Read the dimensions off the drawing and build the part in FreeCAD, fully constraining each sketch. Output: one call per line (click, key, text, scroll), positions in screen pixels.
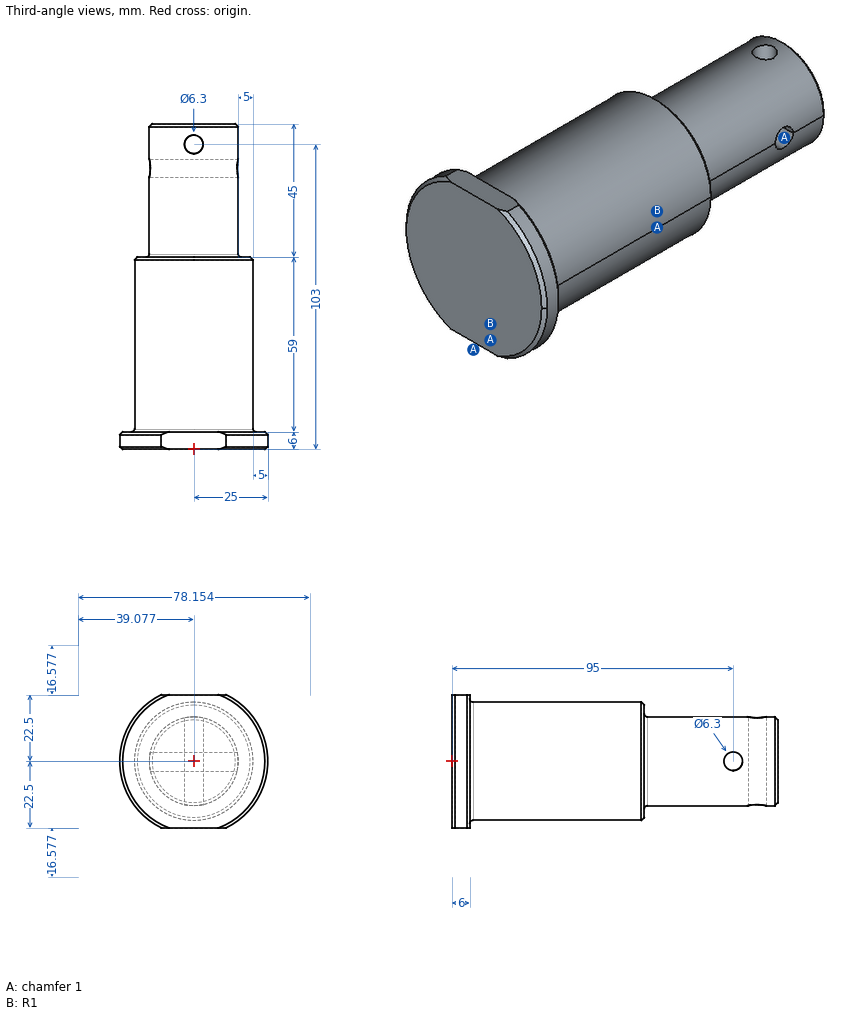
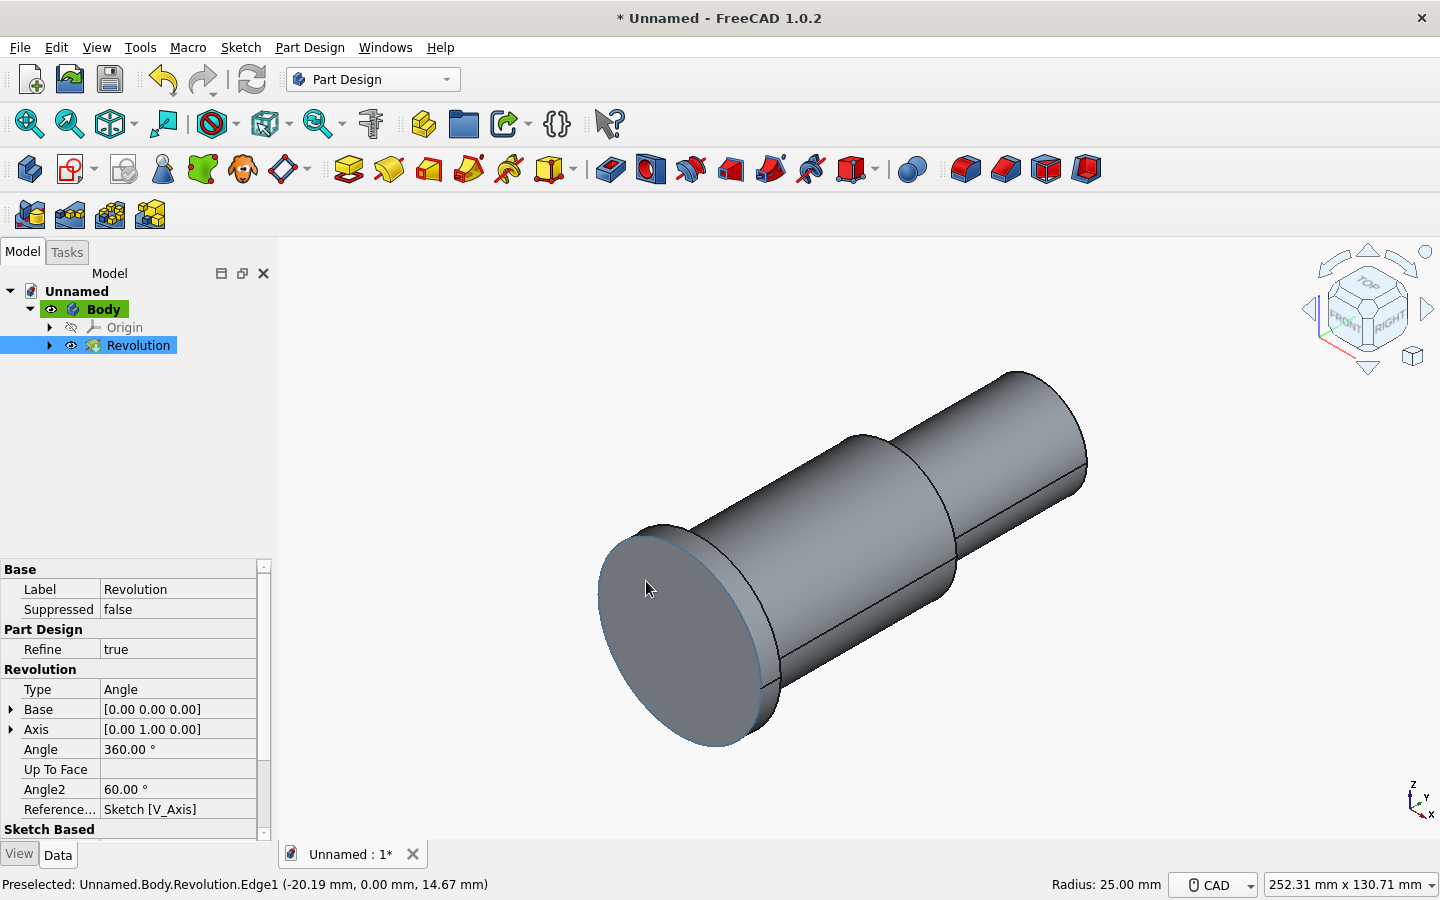
key(2)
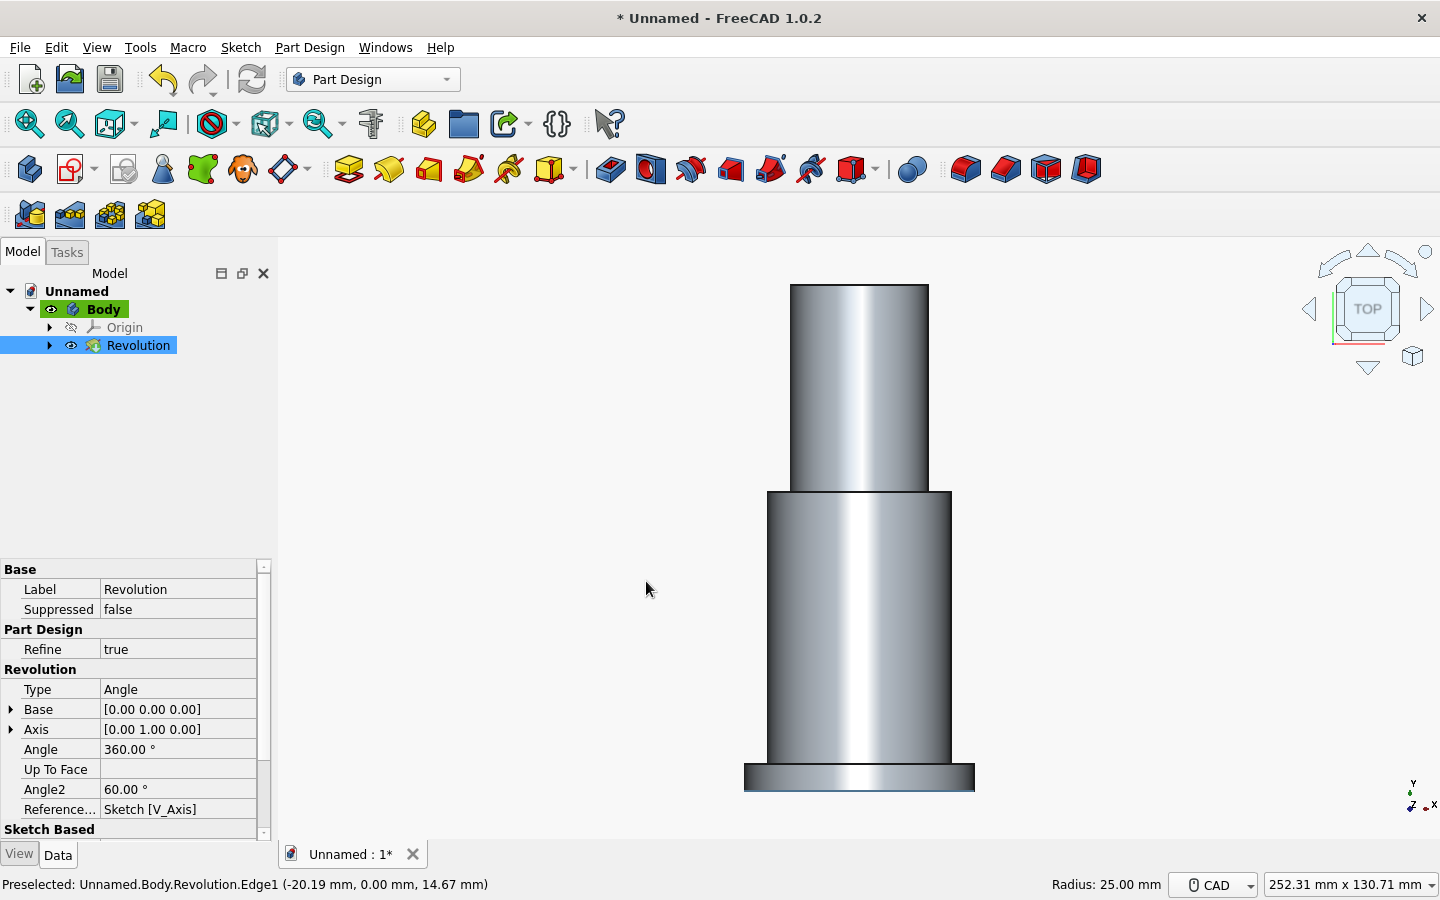
click(803, 284, ctrl)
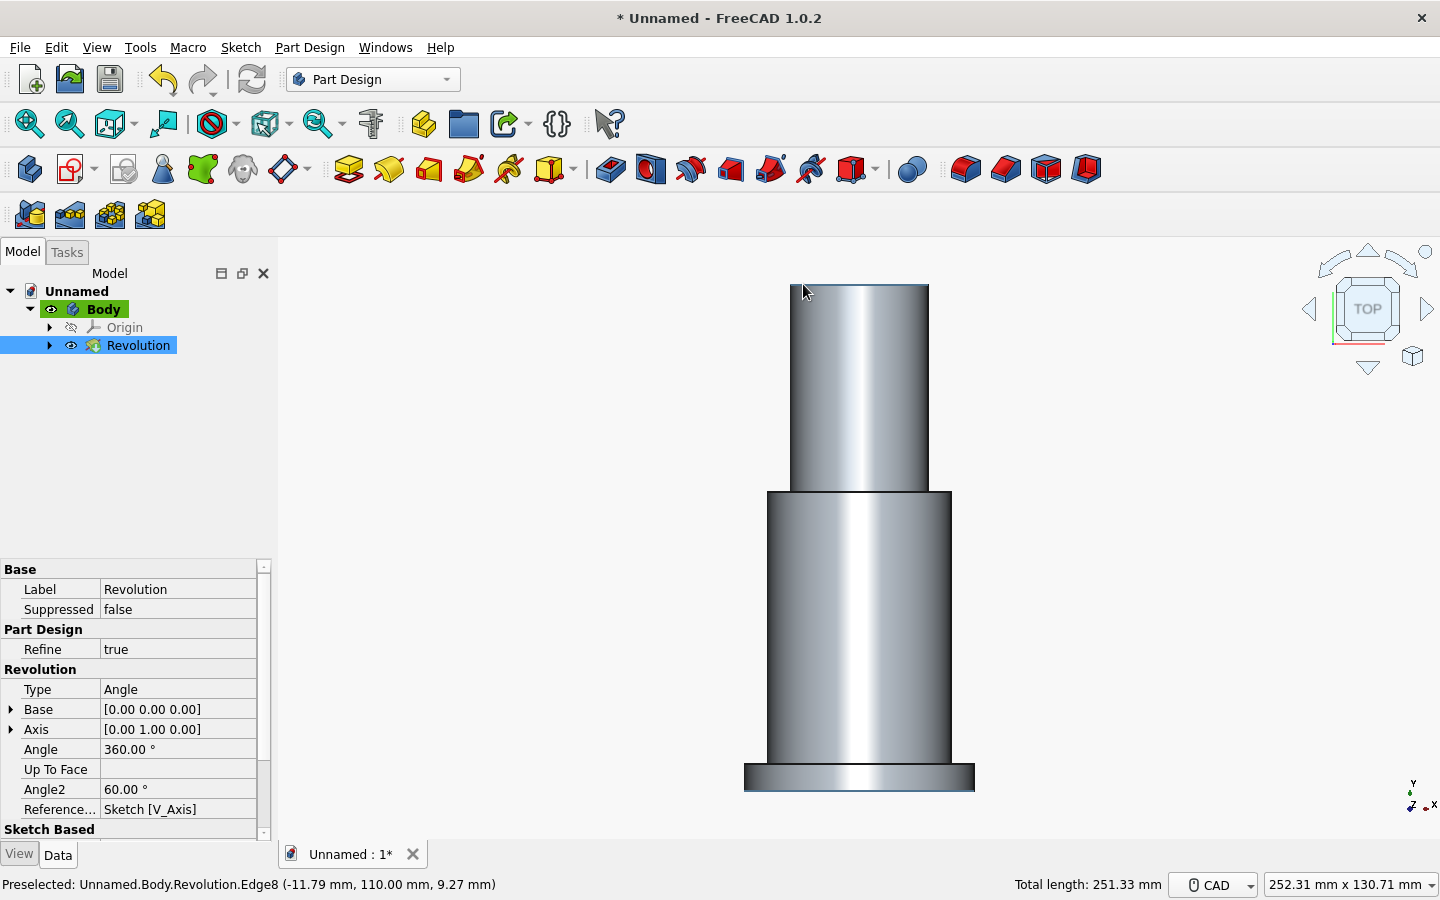
click(784, 491, ctrl)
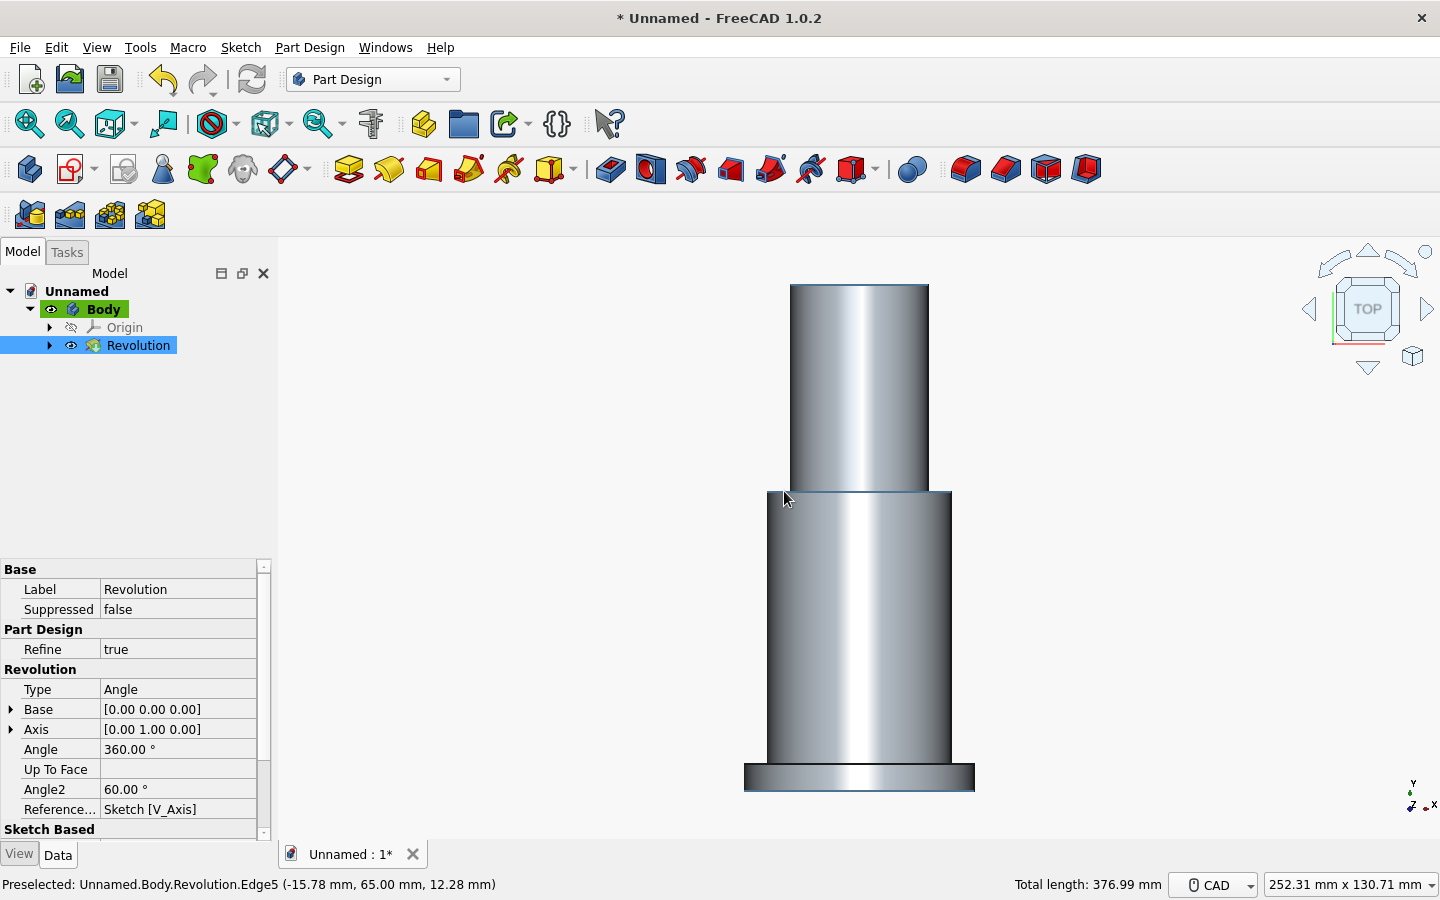
click(766, 763, ctrl)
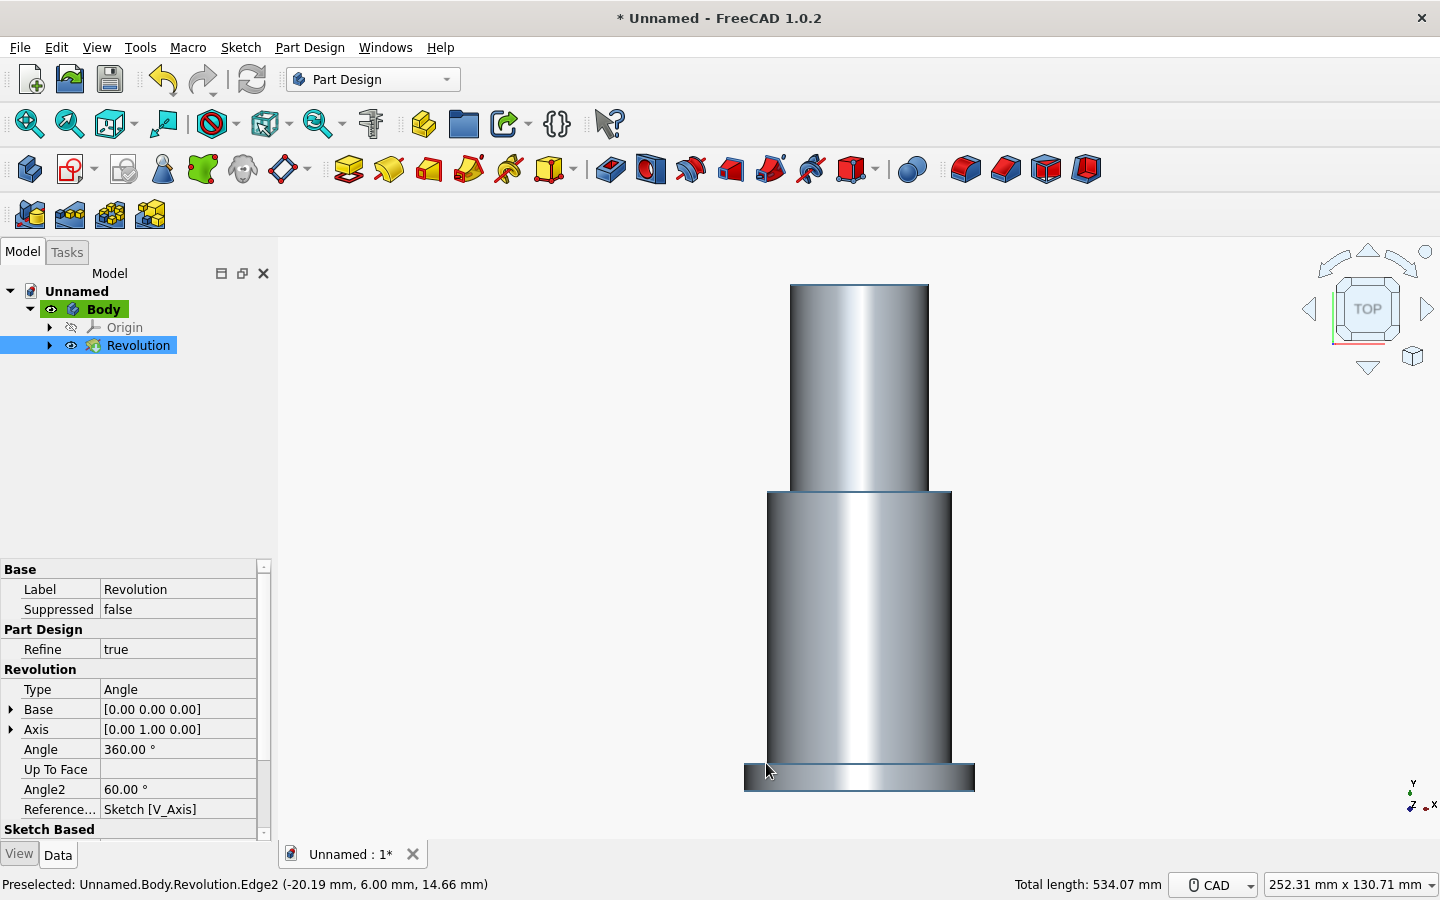
click(1006, 170)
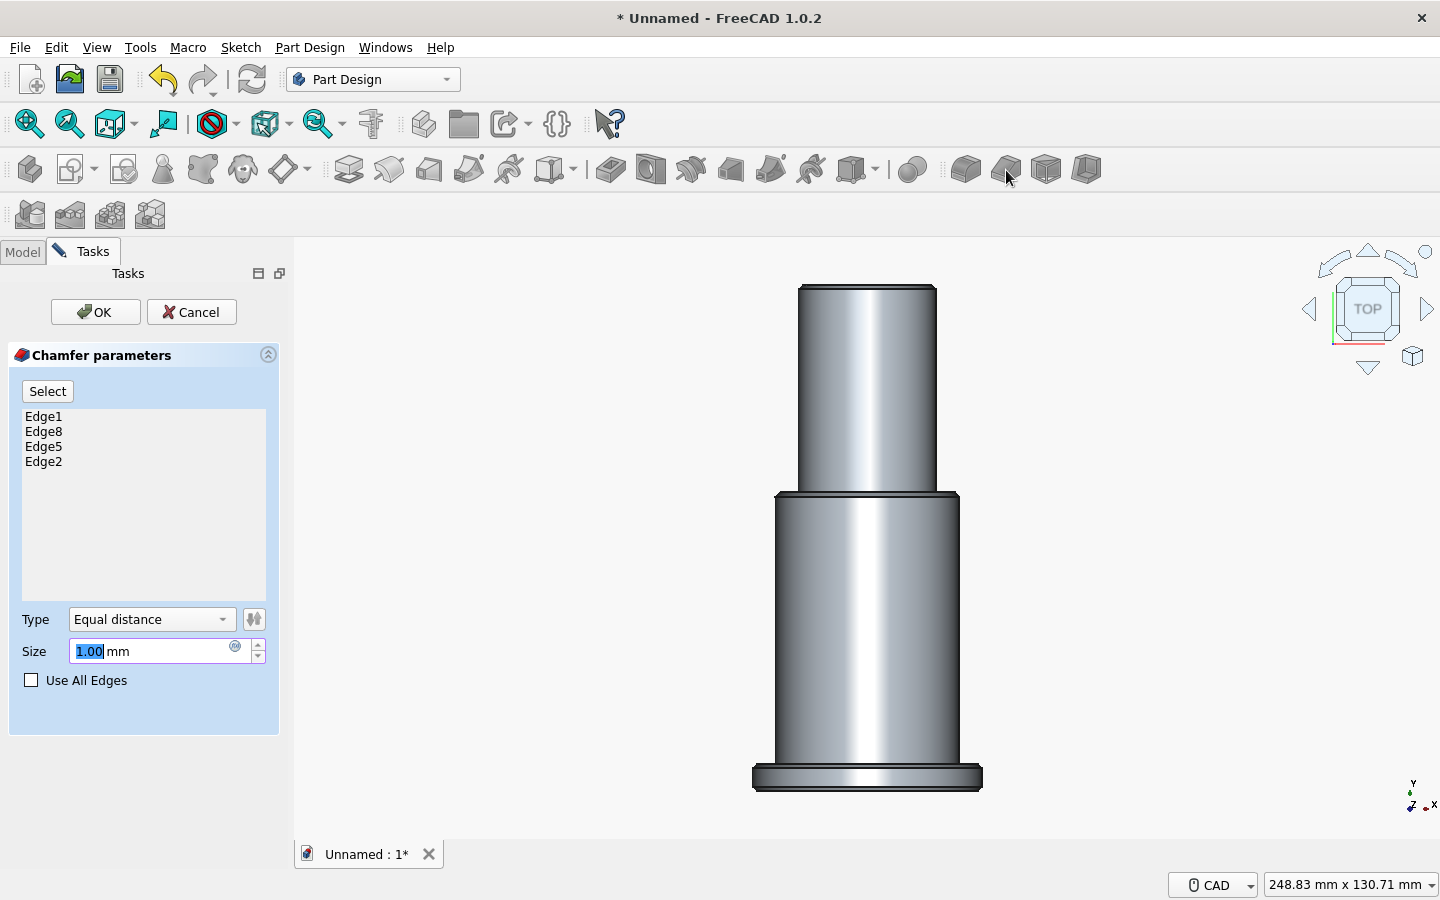
text(1)
key(Tab)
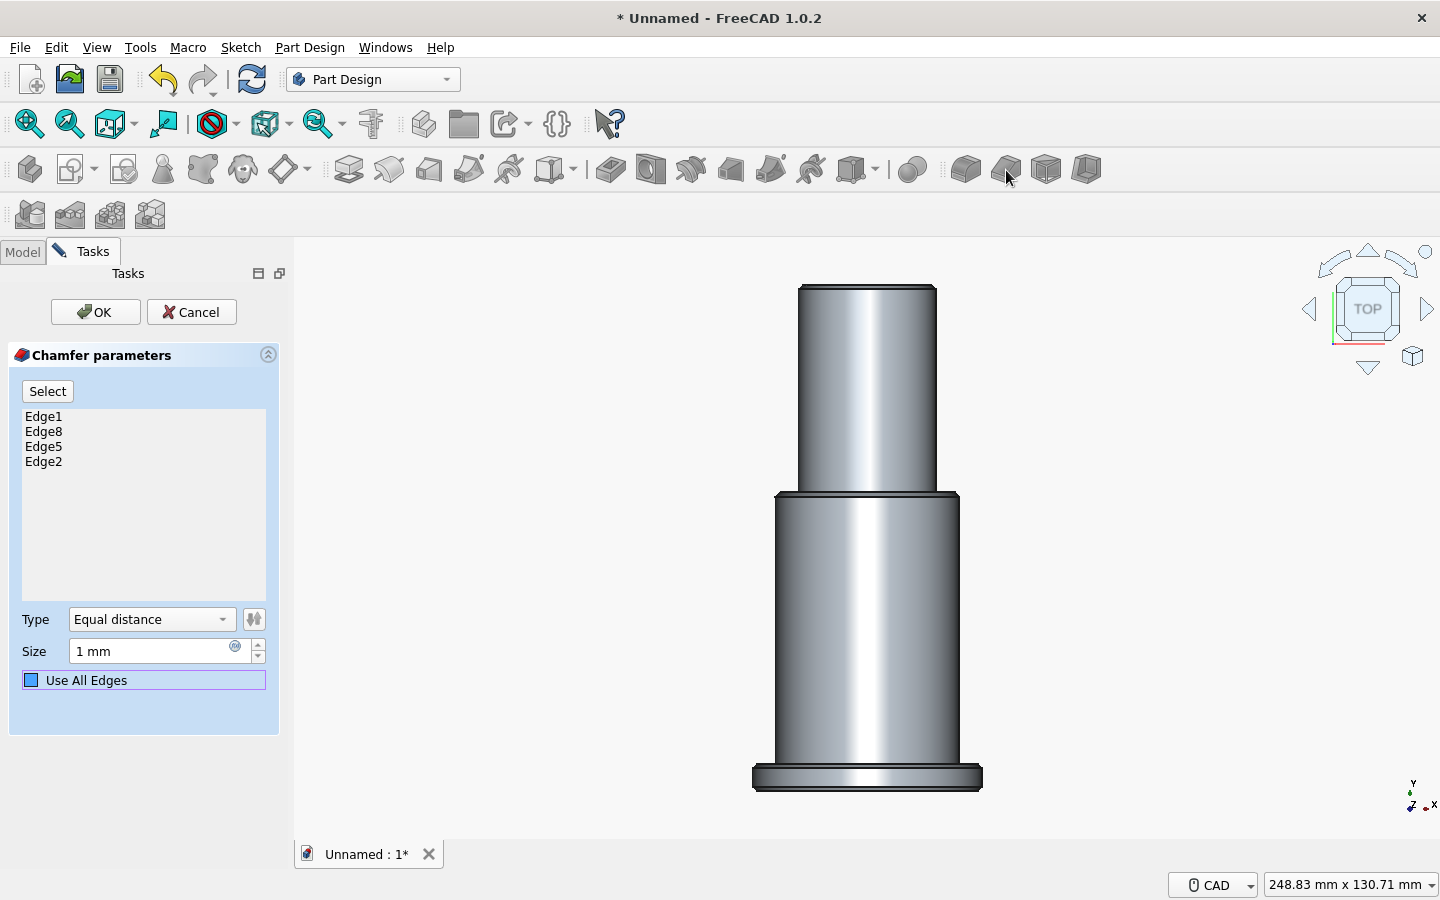
click(96, 312)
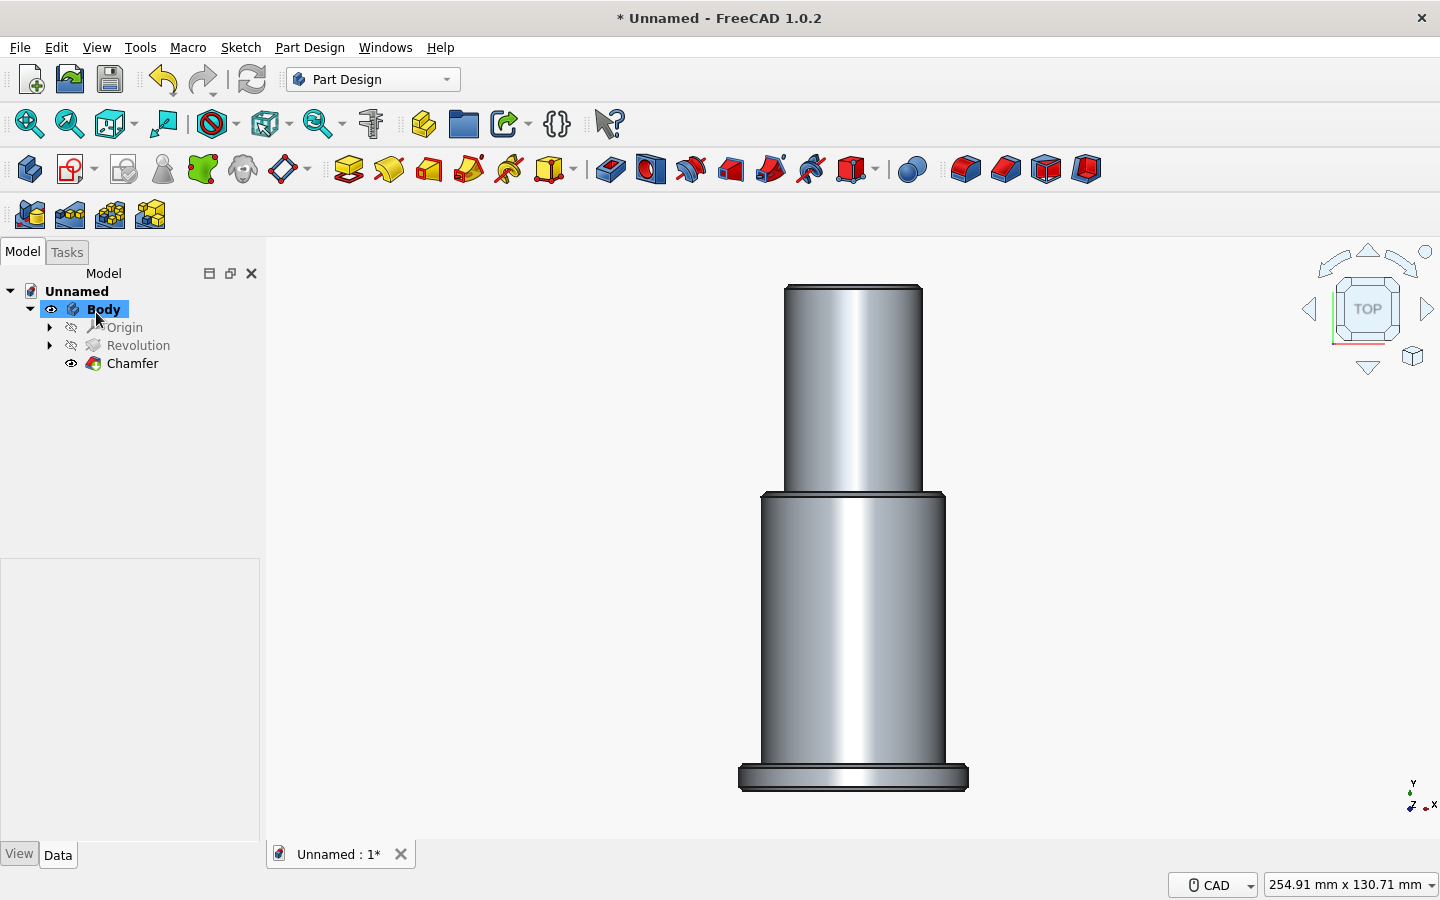
key(0)